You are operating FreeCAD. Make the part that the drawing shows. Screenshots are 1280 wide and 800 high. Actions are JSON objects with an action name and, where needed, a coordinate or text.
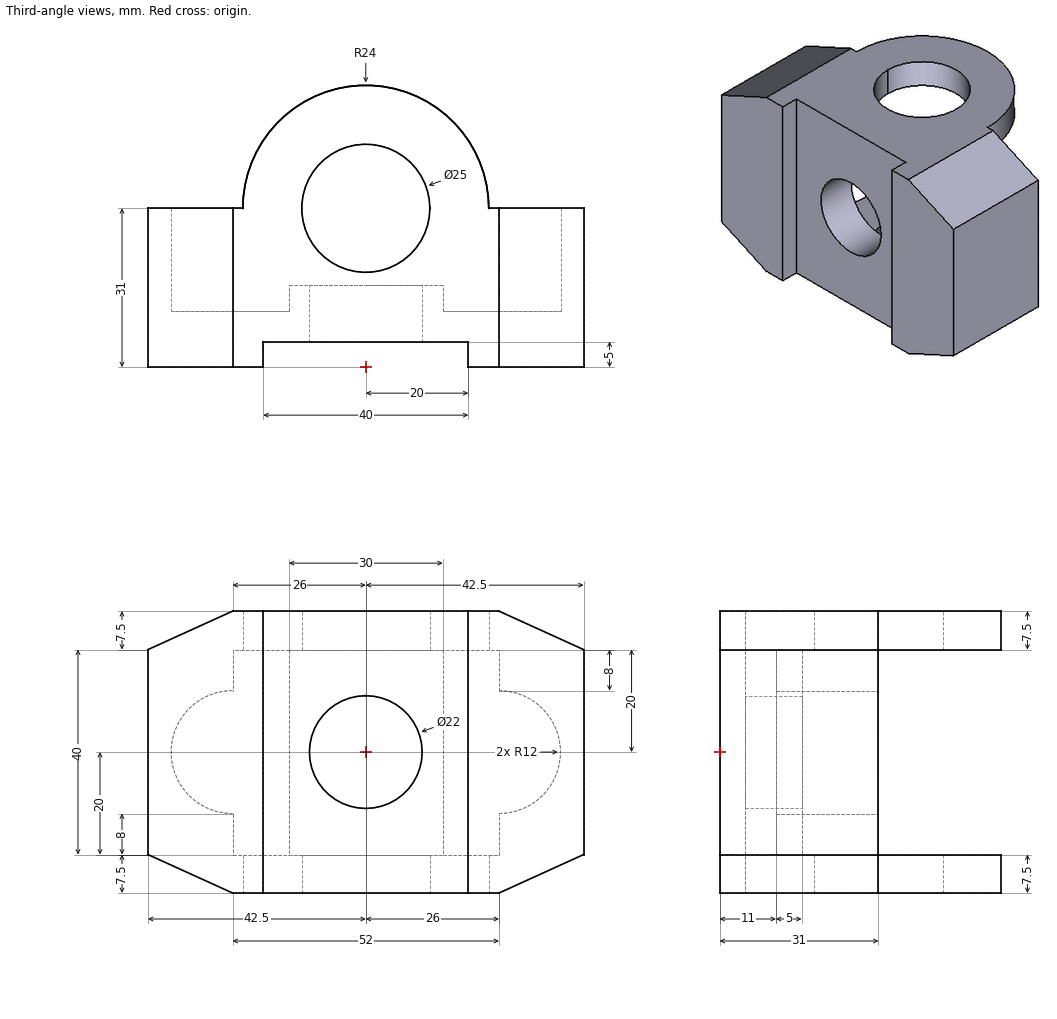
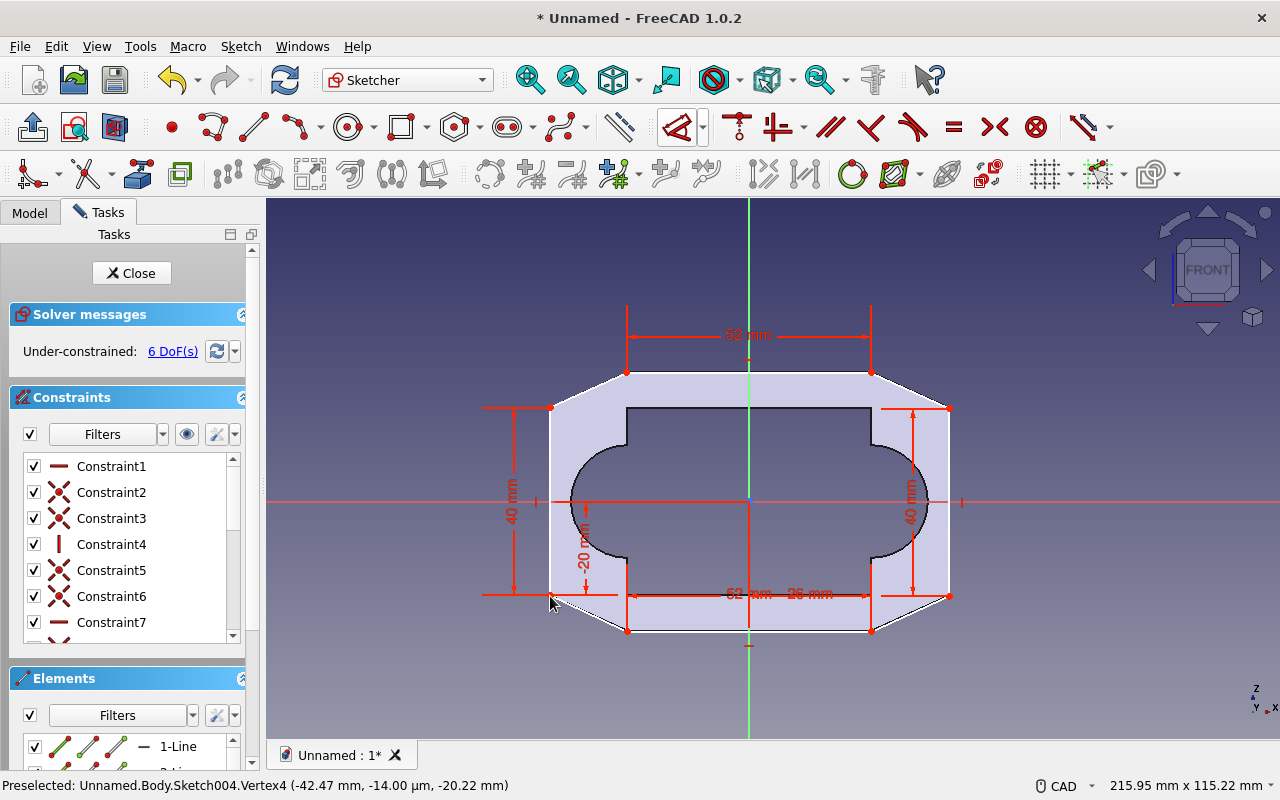
{"action": "left_click", "coordinate": [627, 373]}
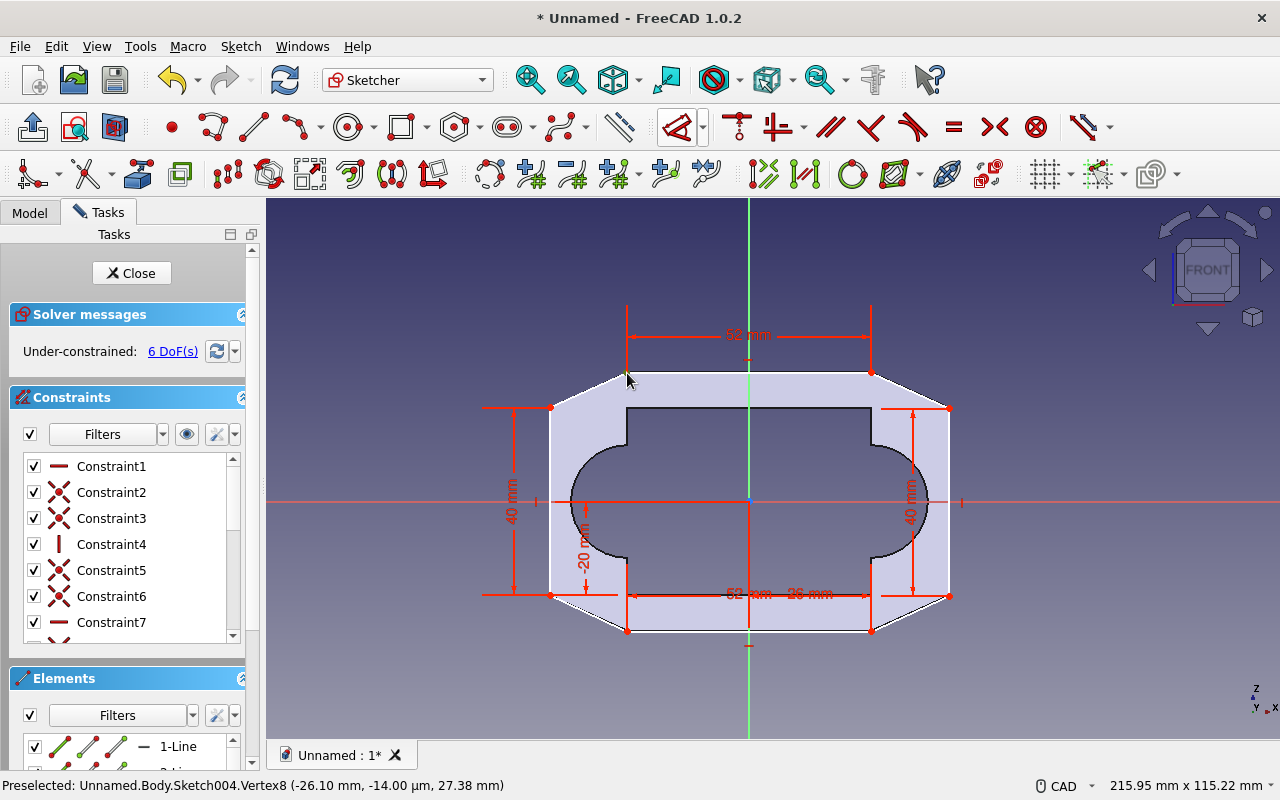
{"action": "left_click", "coordinate": [702, 128]}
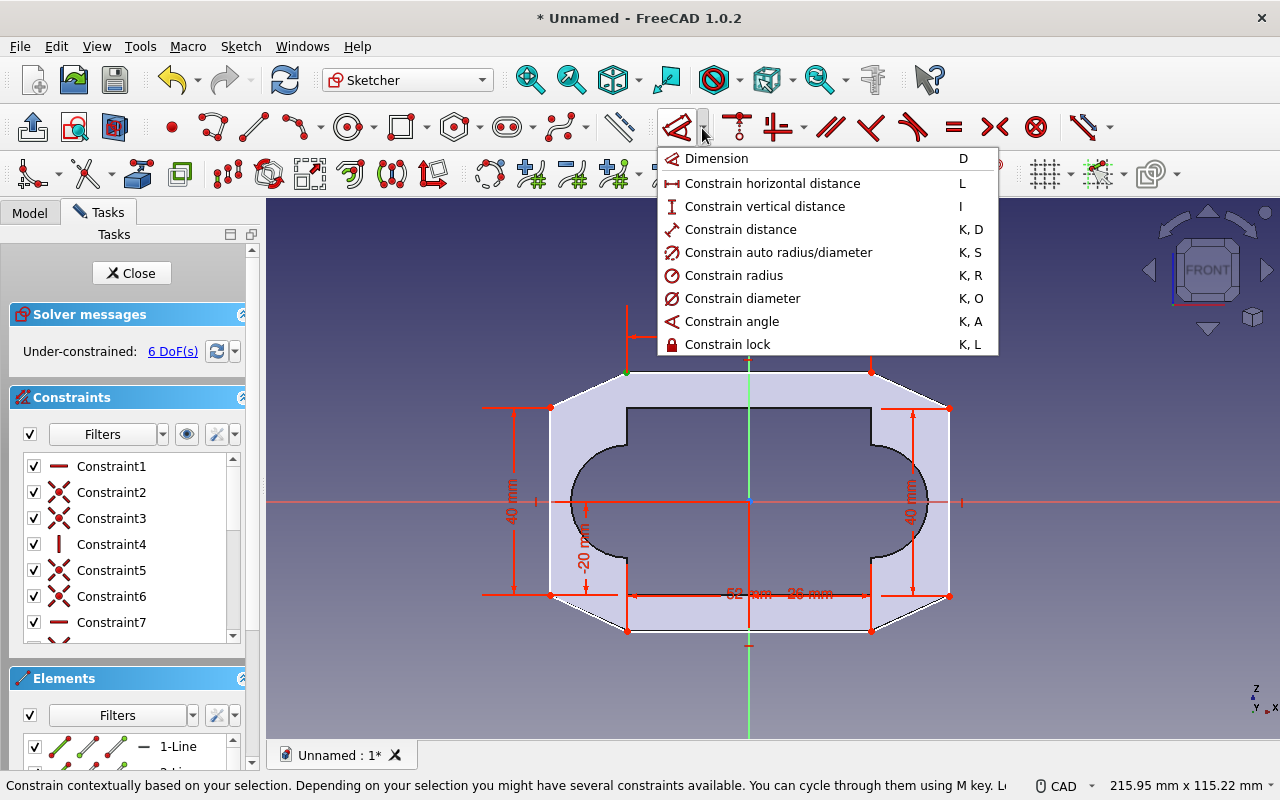
{"action": "left_click", "coordinate": [828, 184]}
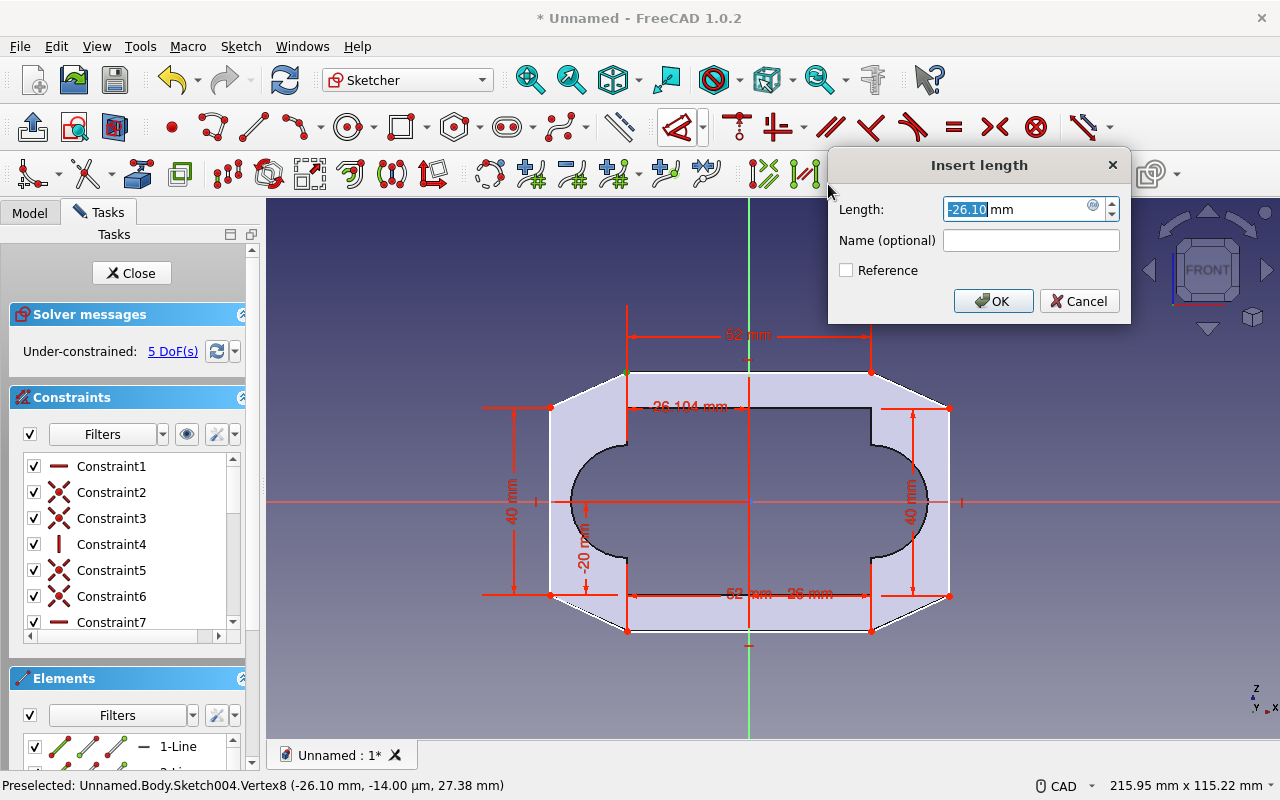
{"action": "type", "text": "-26"}
{"action": "key", "text": "Return"}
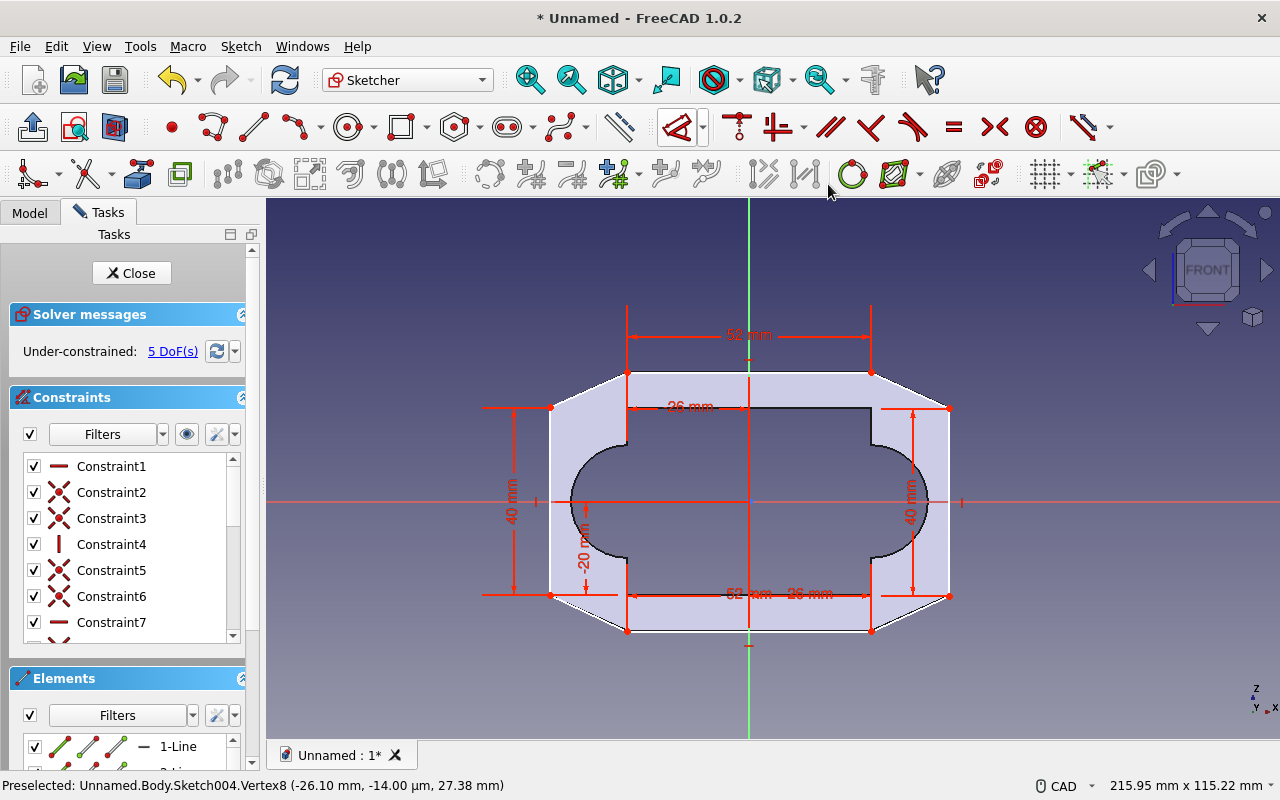
{"action": "left_click", "coordinate": [949, 409]}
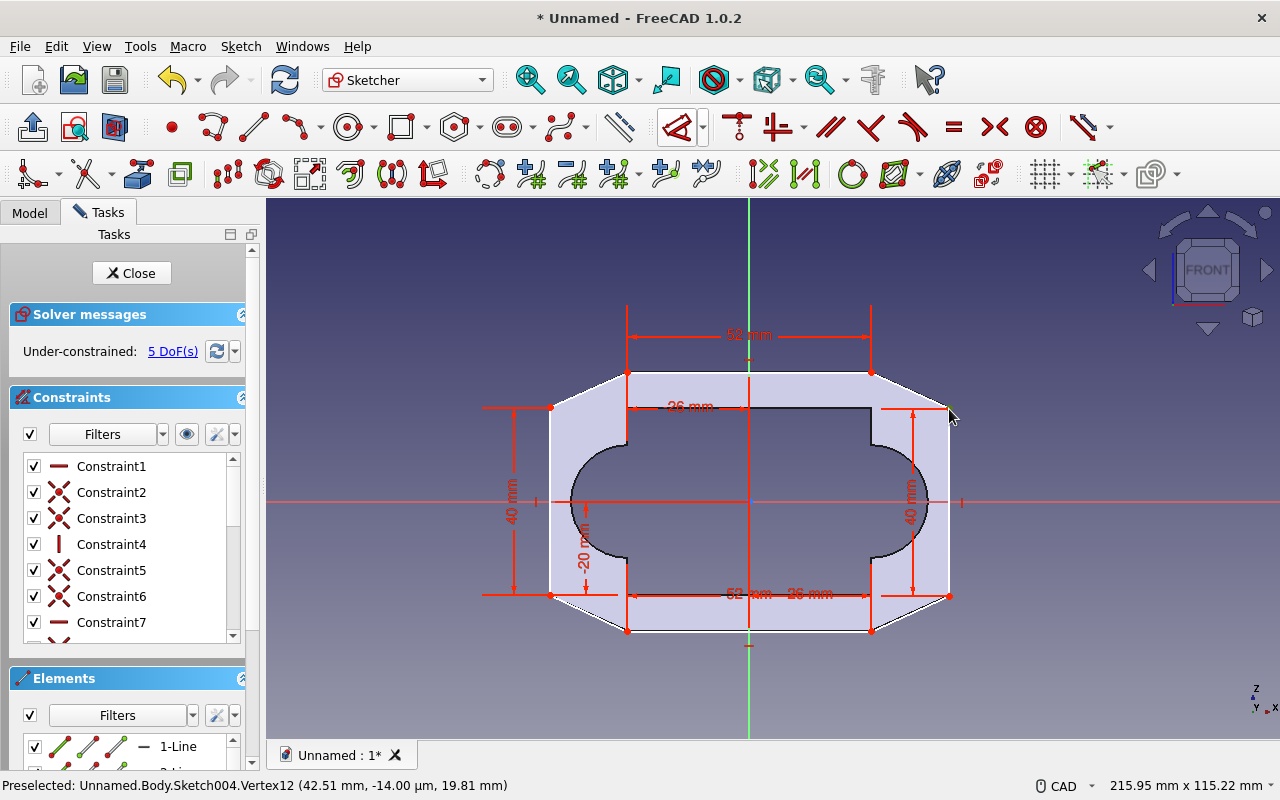
{"action": "left_click", "coordinate": [702, 128]}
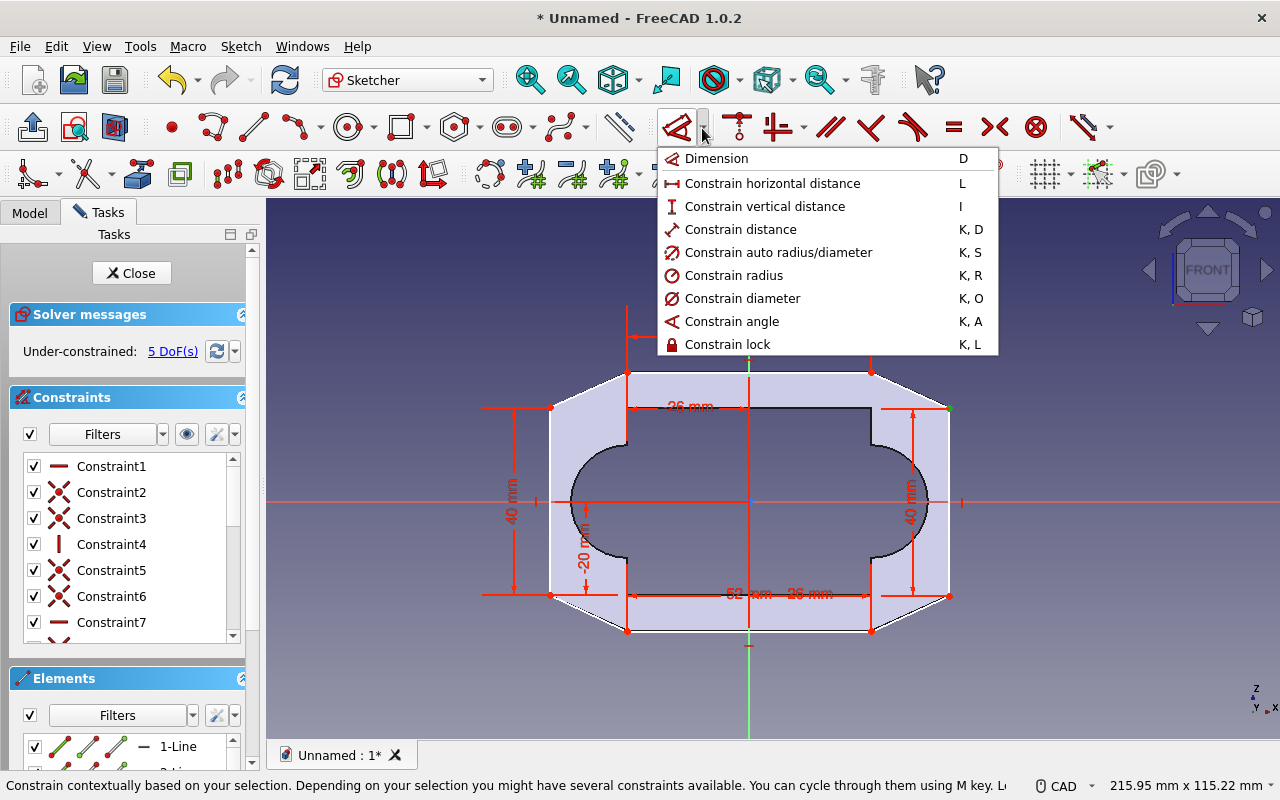
{"action": "left_click", "coordinate": [828, 206]}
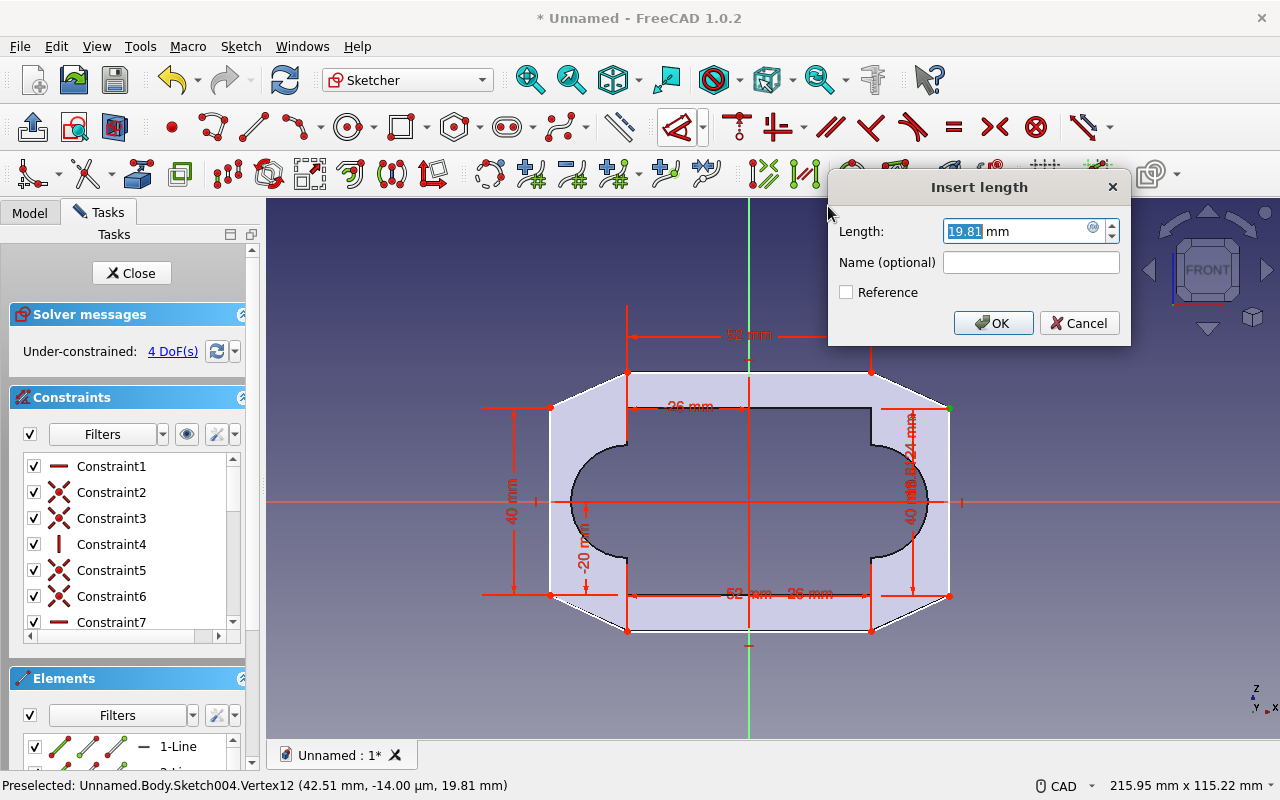
{"action": "type", "text": "20"}
{"action": "key", "text": "Return"}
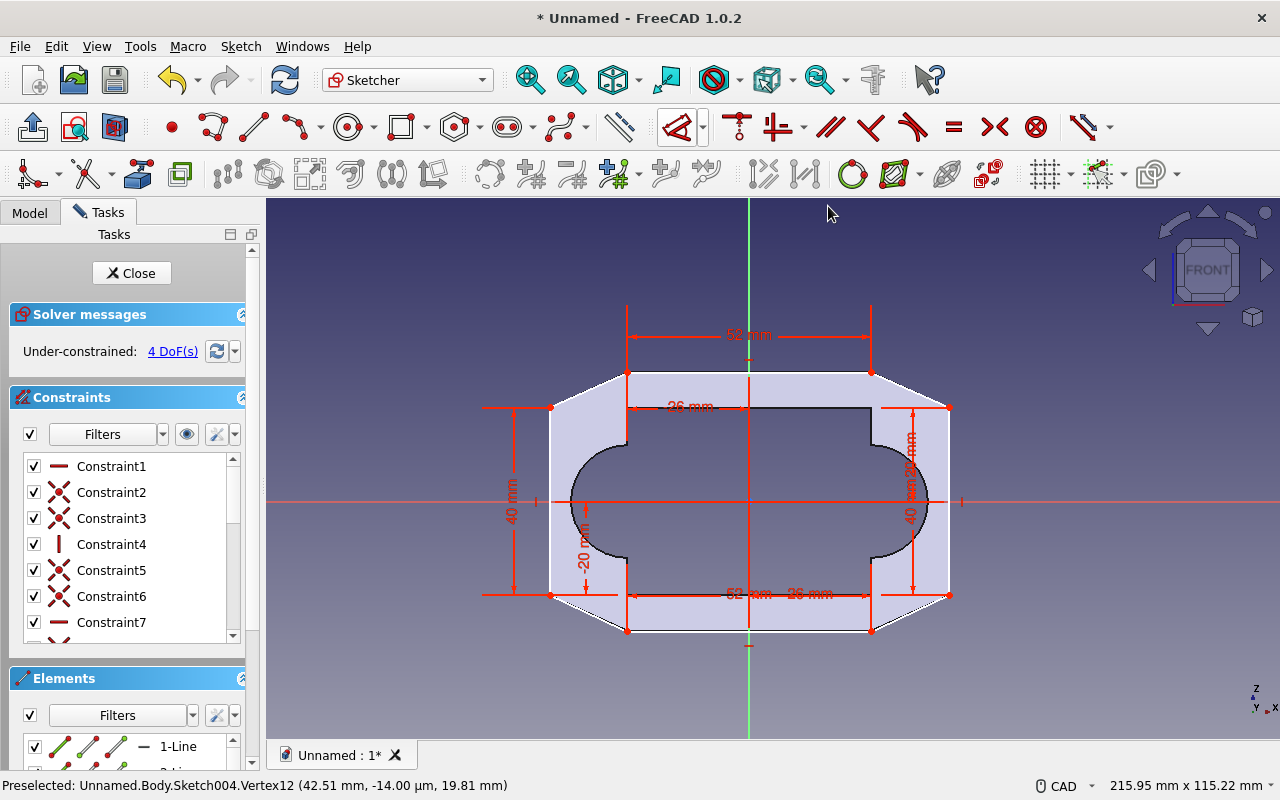
{"action": "left_click", "coordinate": [604, 621]}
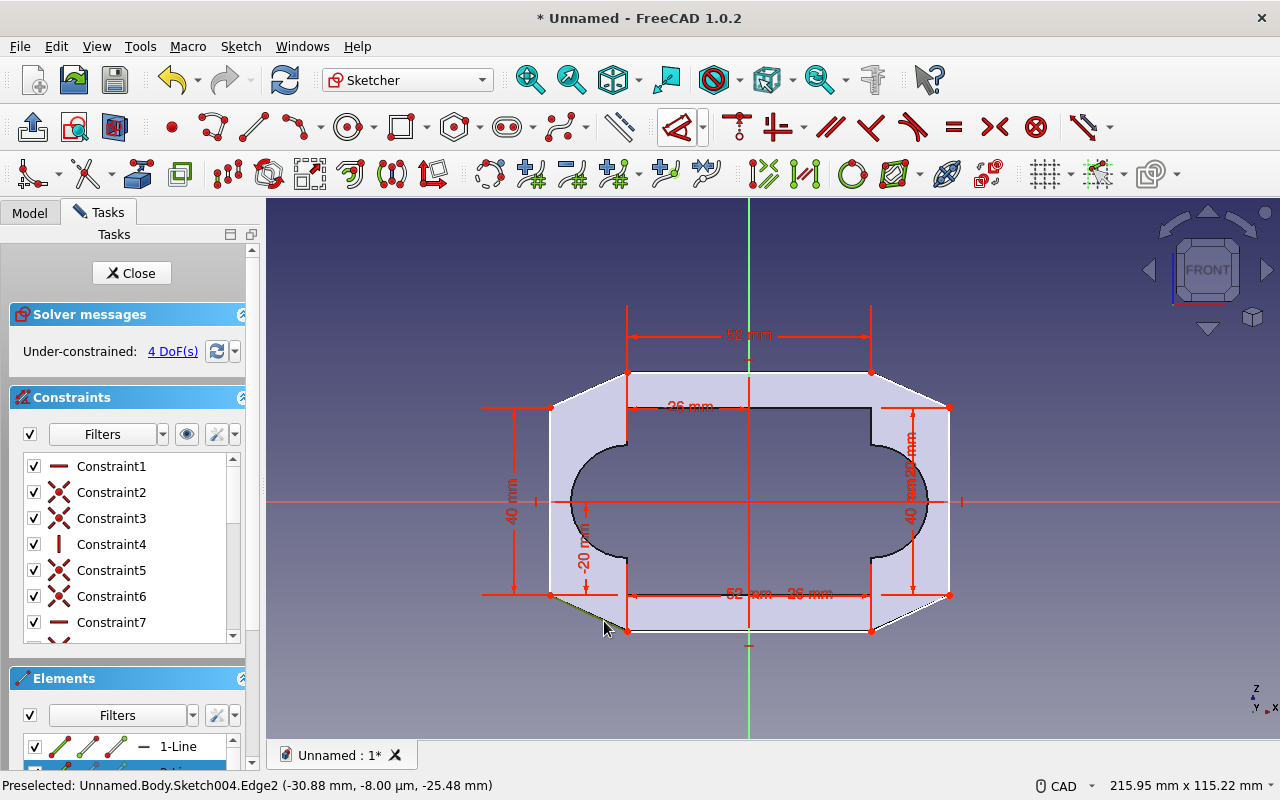
{"action": "left_click", "coordinate": [702, 128]}